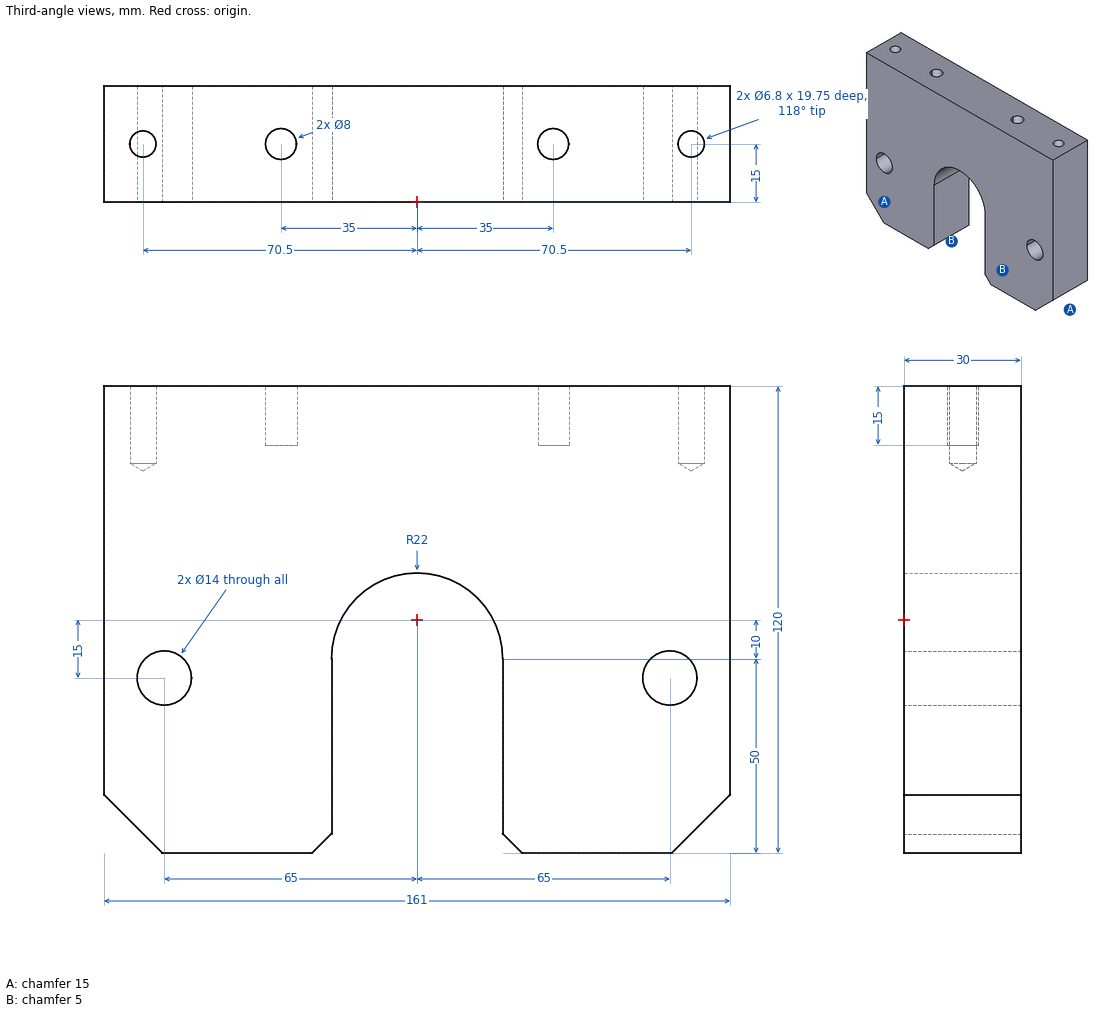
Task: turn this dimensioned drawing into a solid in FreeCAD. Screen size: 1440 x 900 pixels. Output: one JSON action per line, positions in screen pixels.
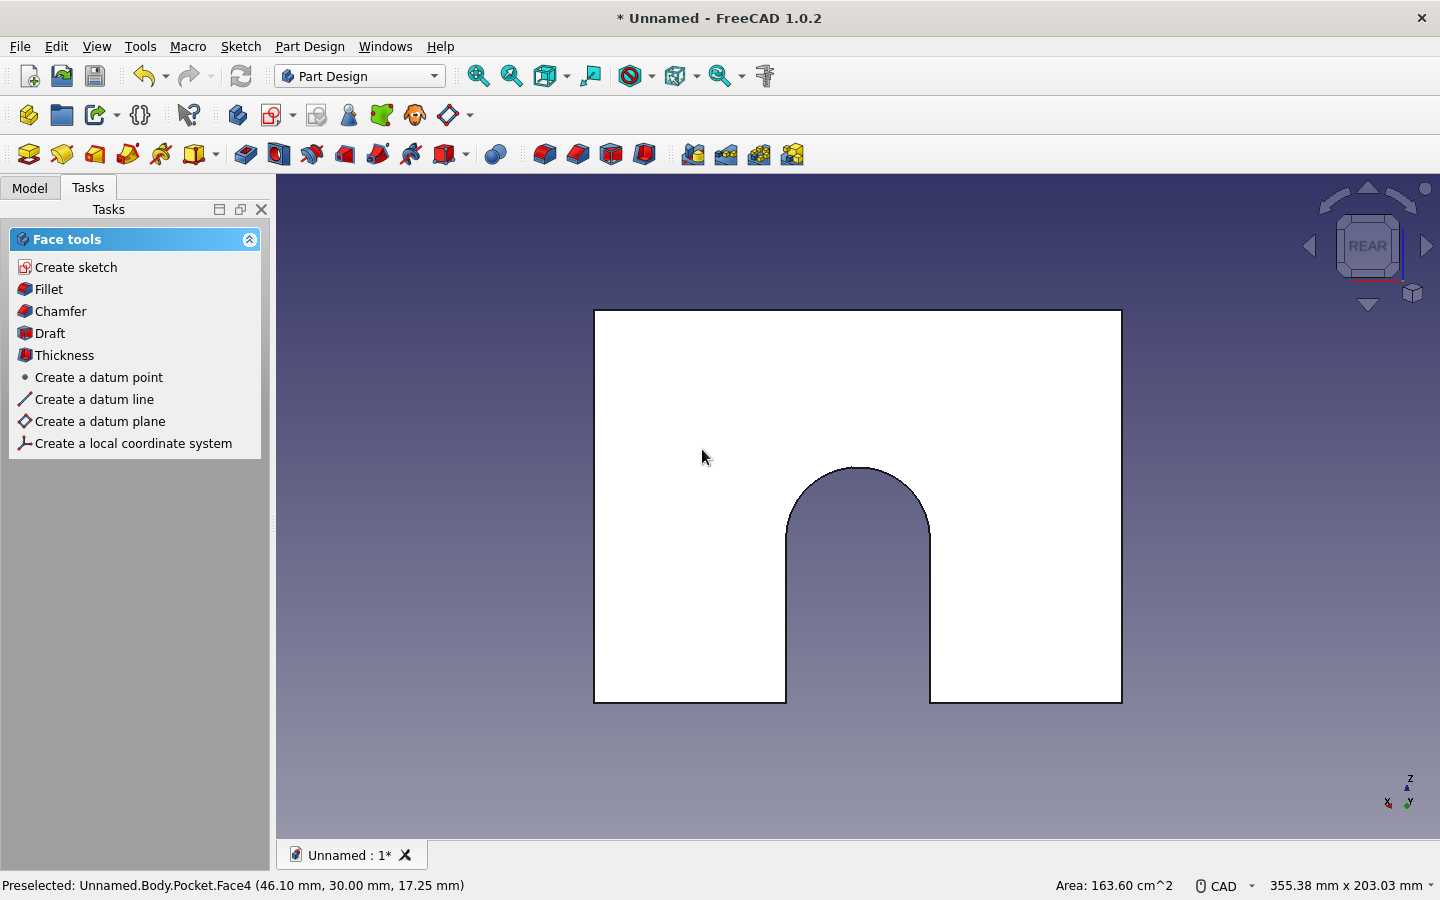
{"action": "left_click", "coordinate": [270, 116]}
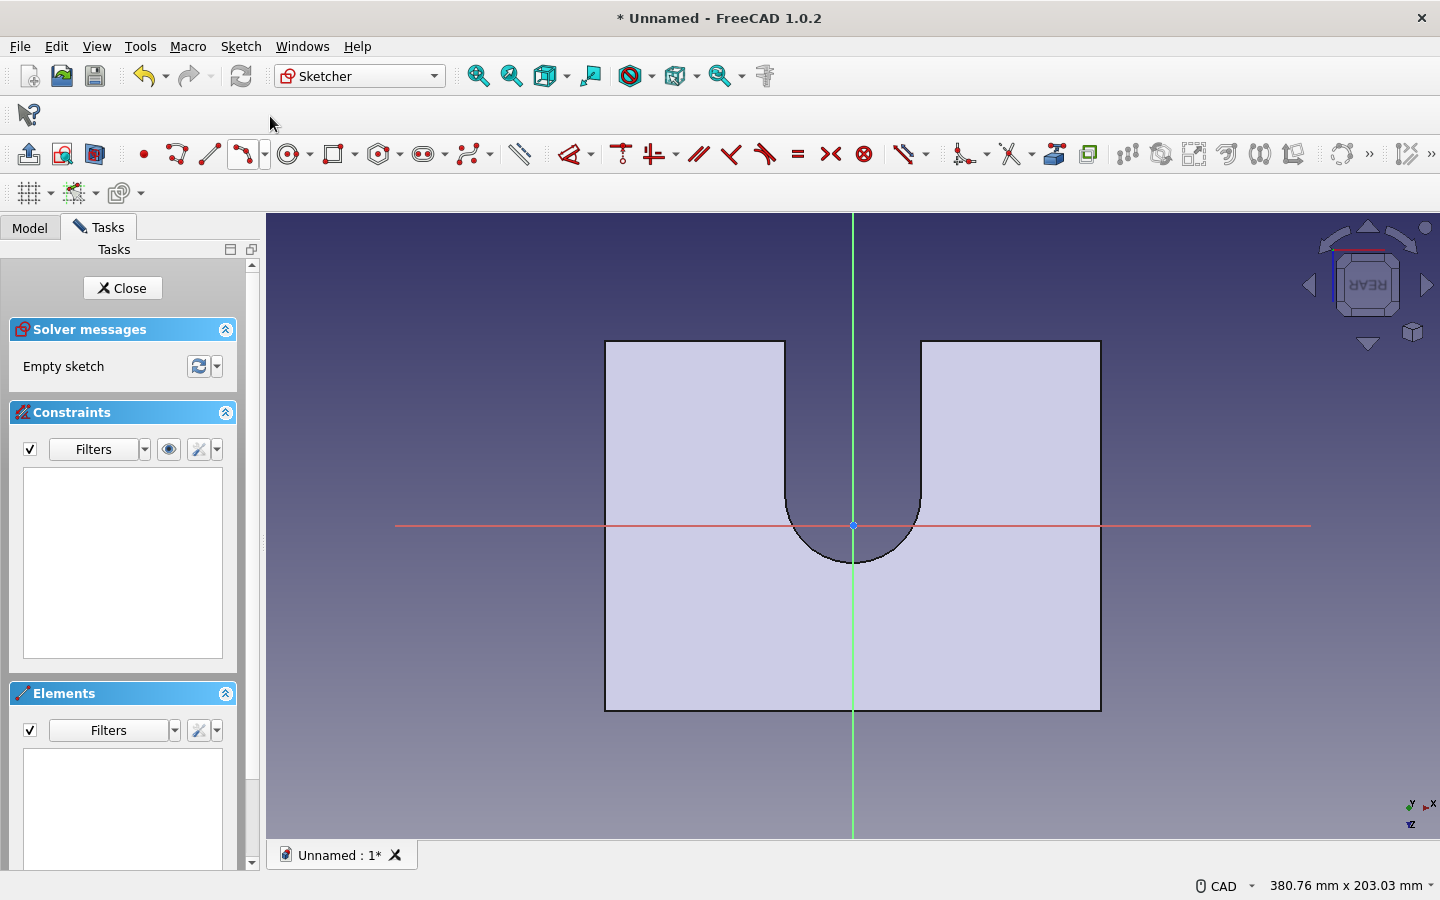
{"action": "scroll", "coordinate": [992, 423], "scroll_direction": "up", "scroll_amount": 2}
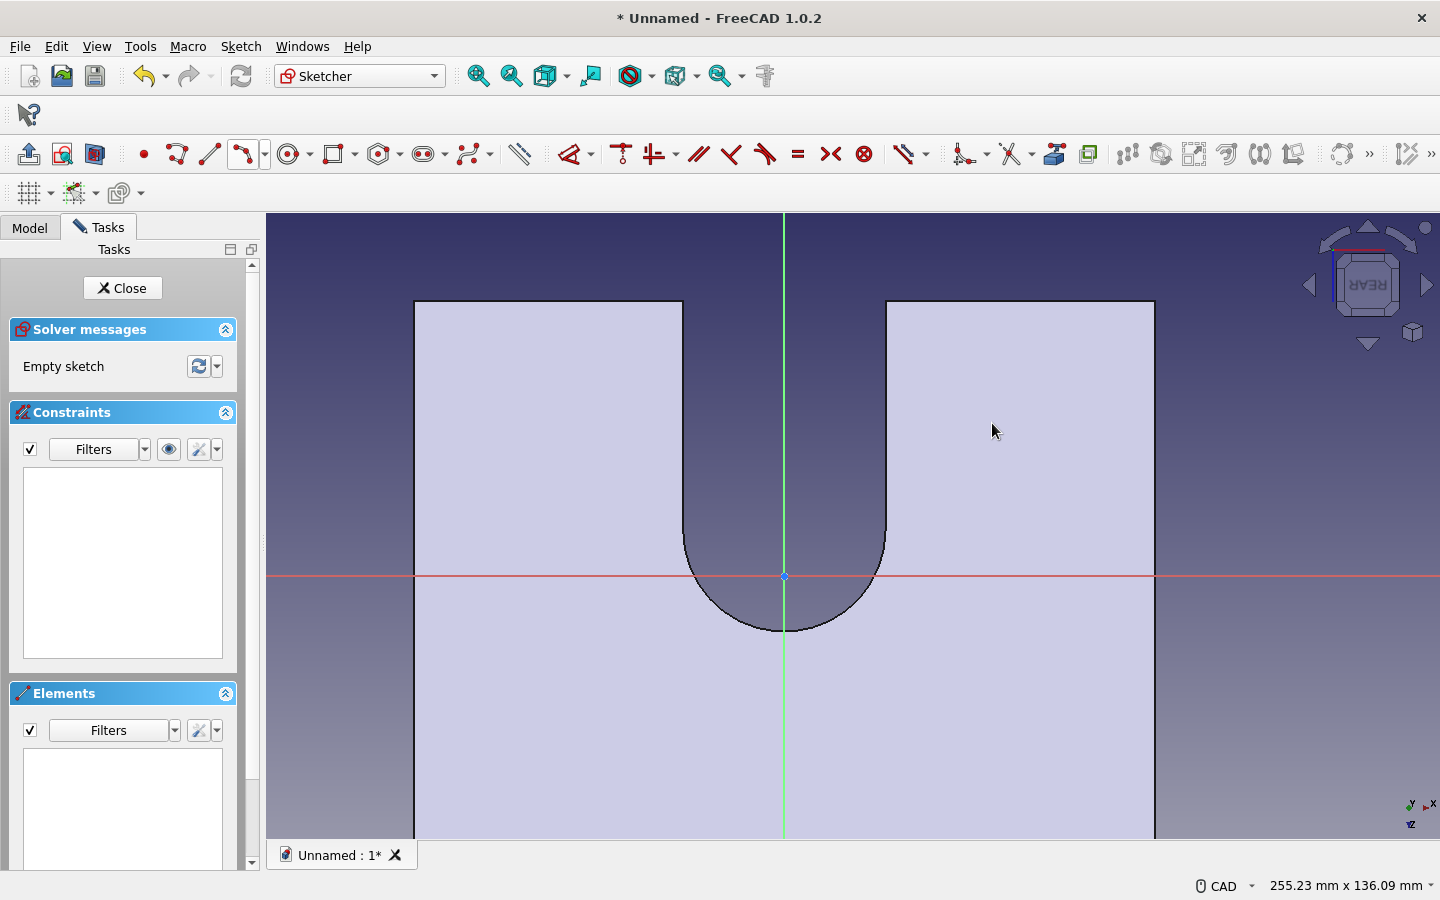
{"action": "key", "text": "g c"}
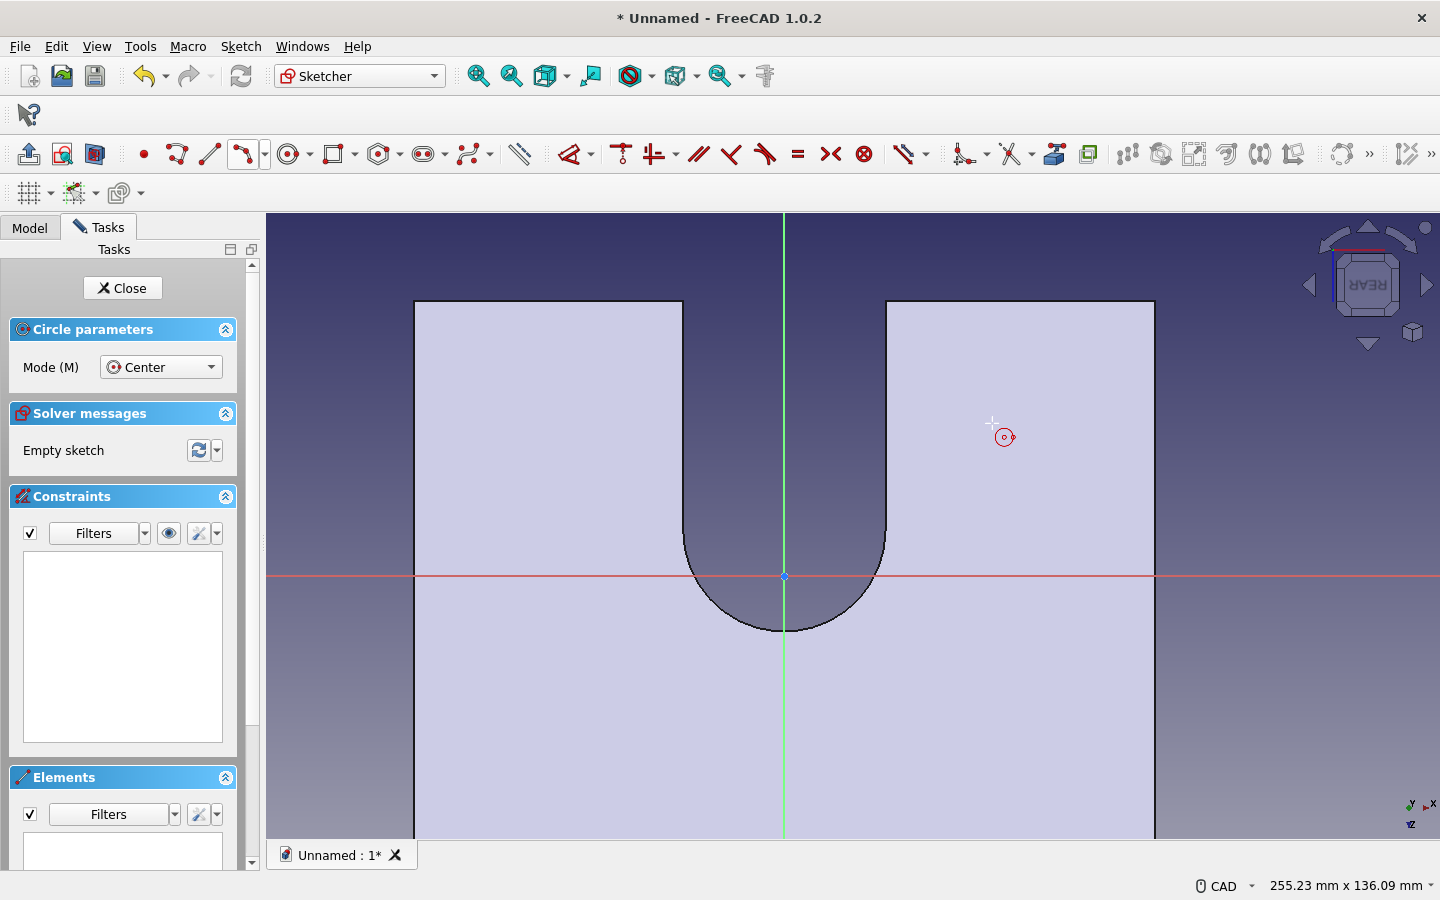
{"action": "left_click", "coordinate": [485, 507]}
{"action": "left_click", "coordinate": [508, 485]}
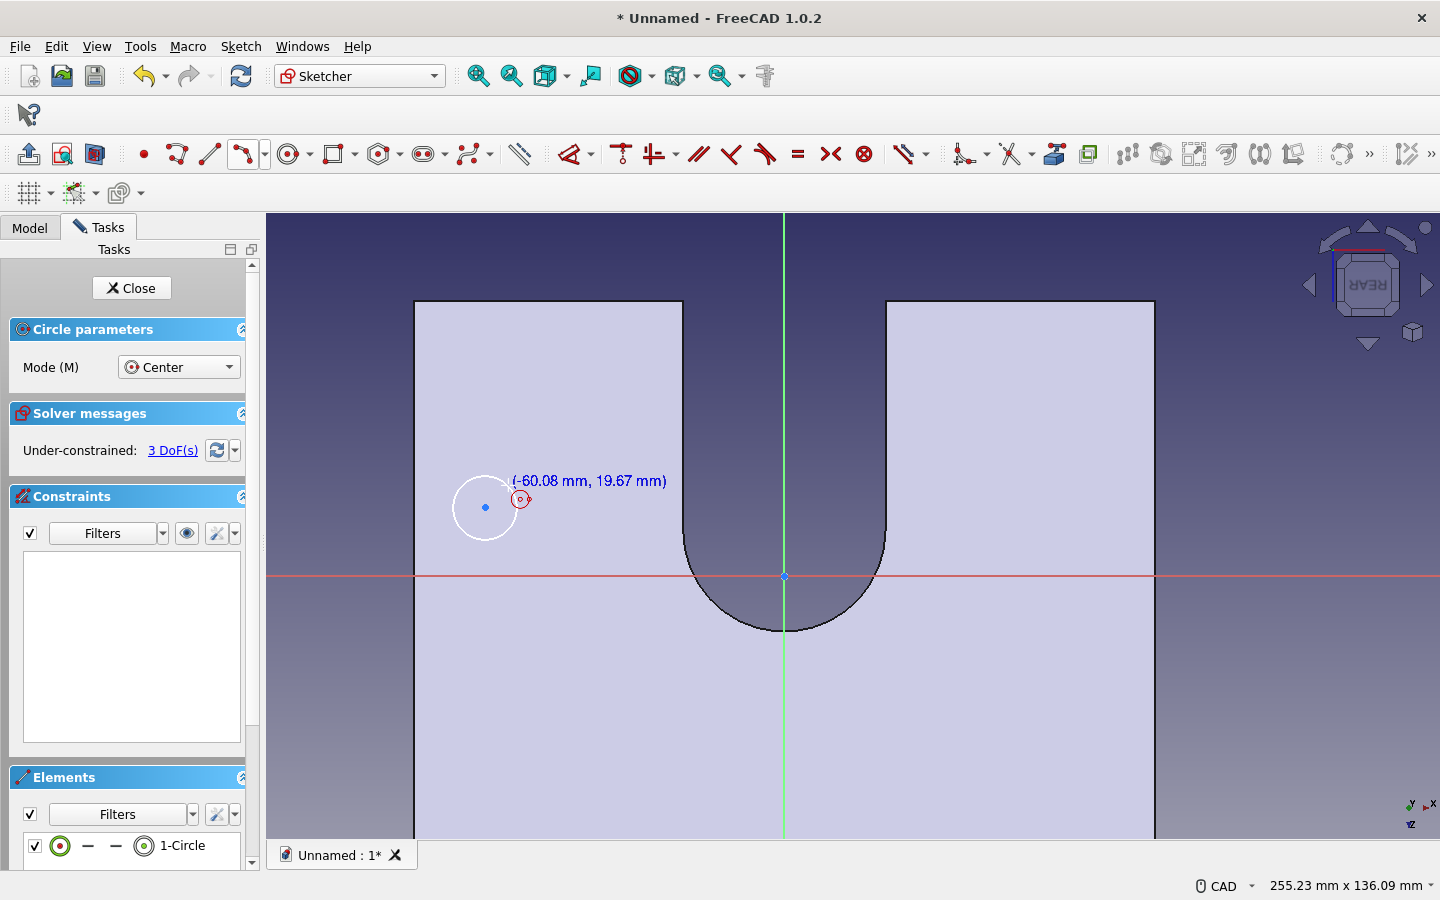
{"action": "left_click", "coordinate": [1083, 507]}
{"action": "left_click", "coordinate": [1106, 485]}
{"action": "key", "text": "Escape"}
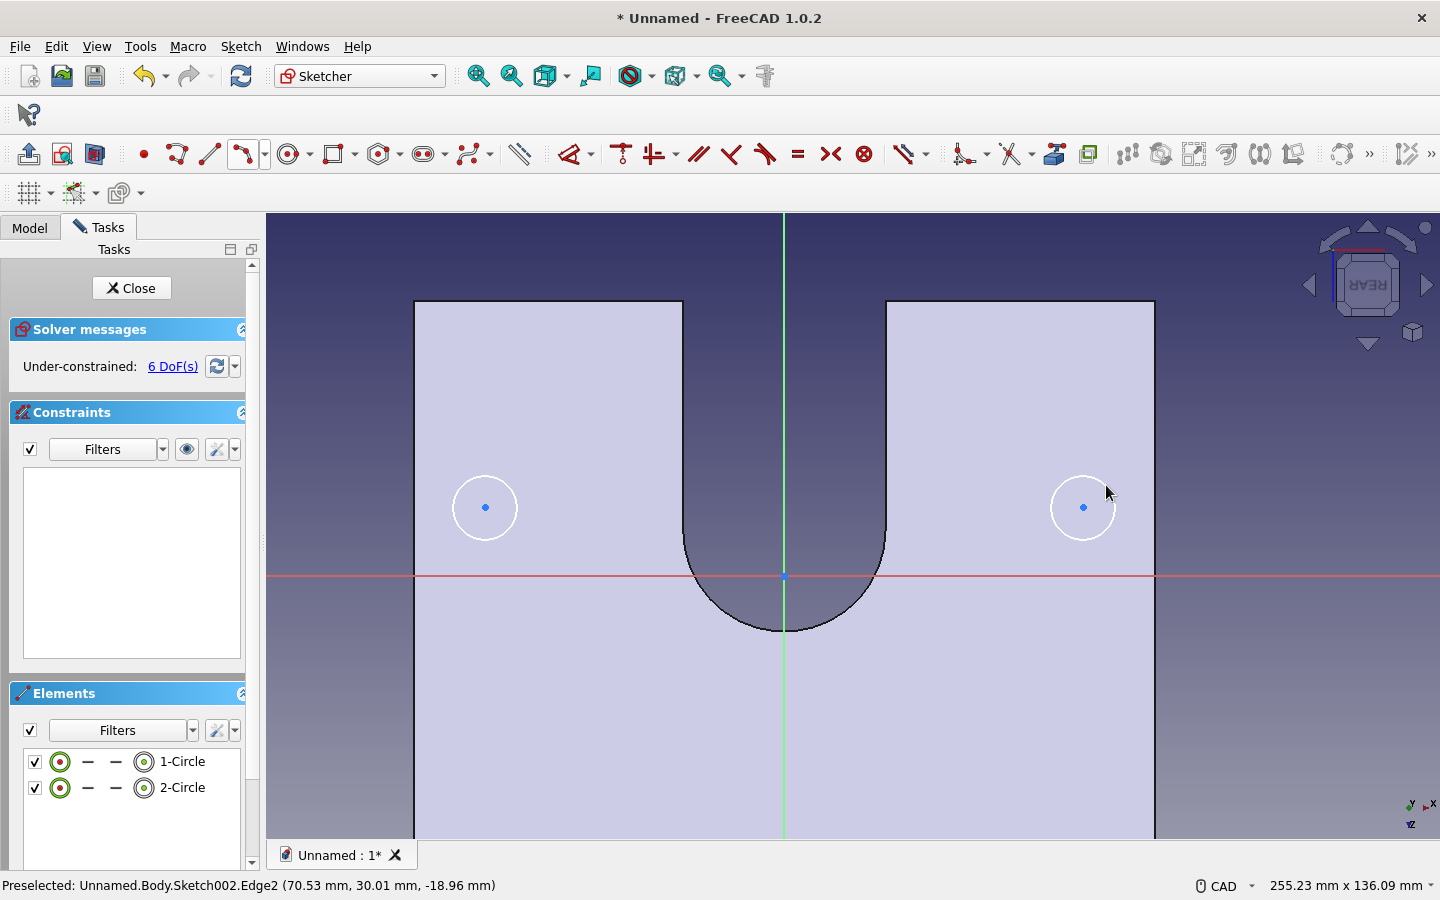
{"action": "left_click", "coordinate": [507, 485]}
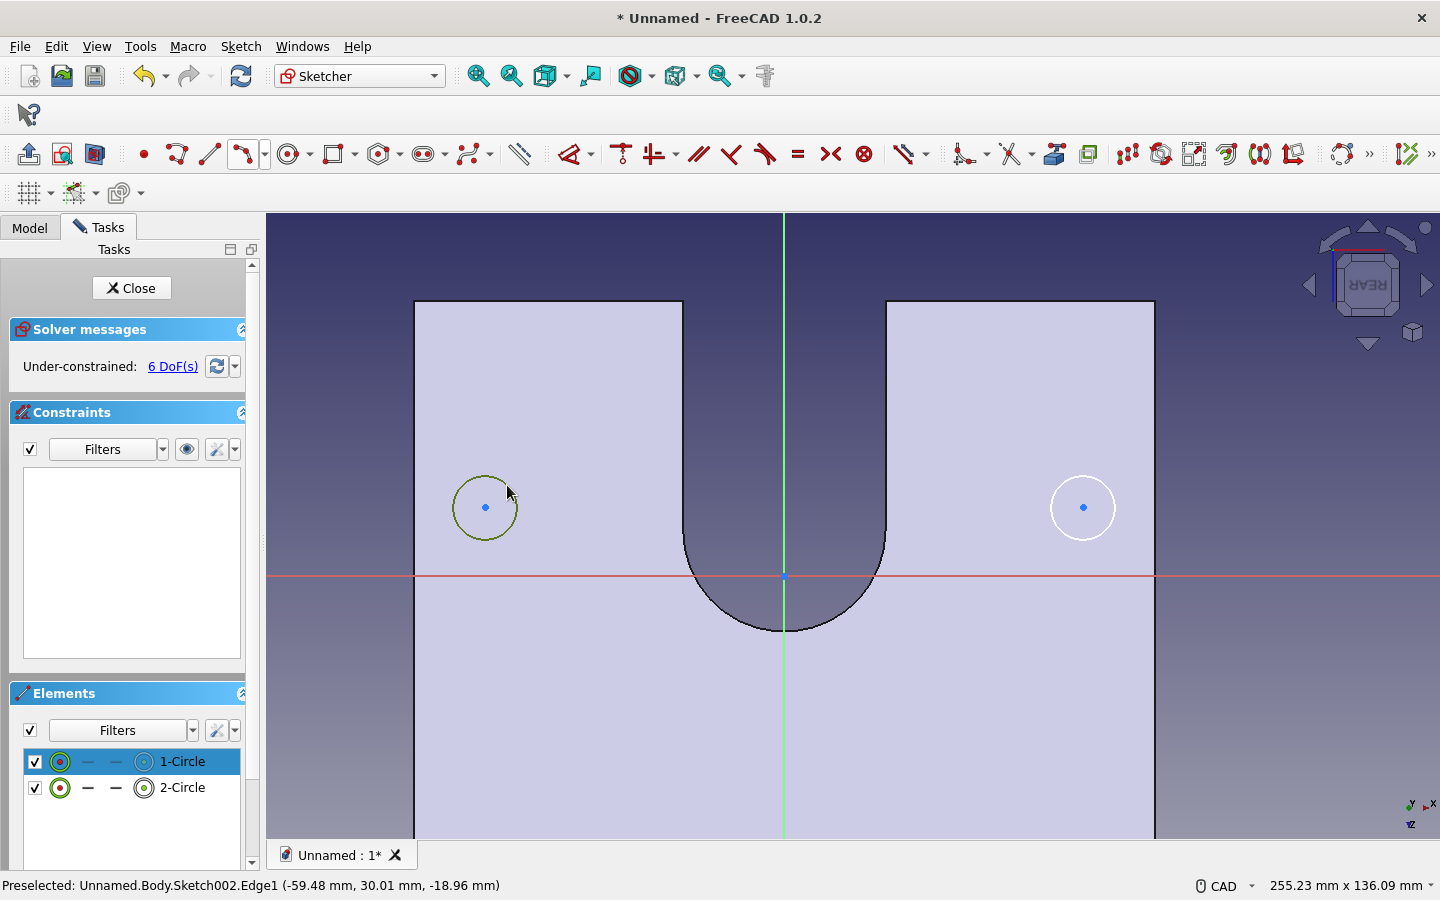
{"action": "left_click", "coordinate": [1105, 485]}